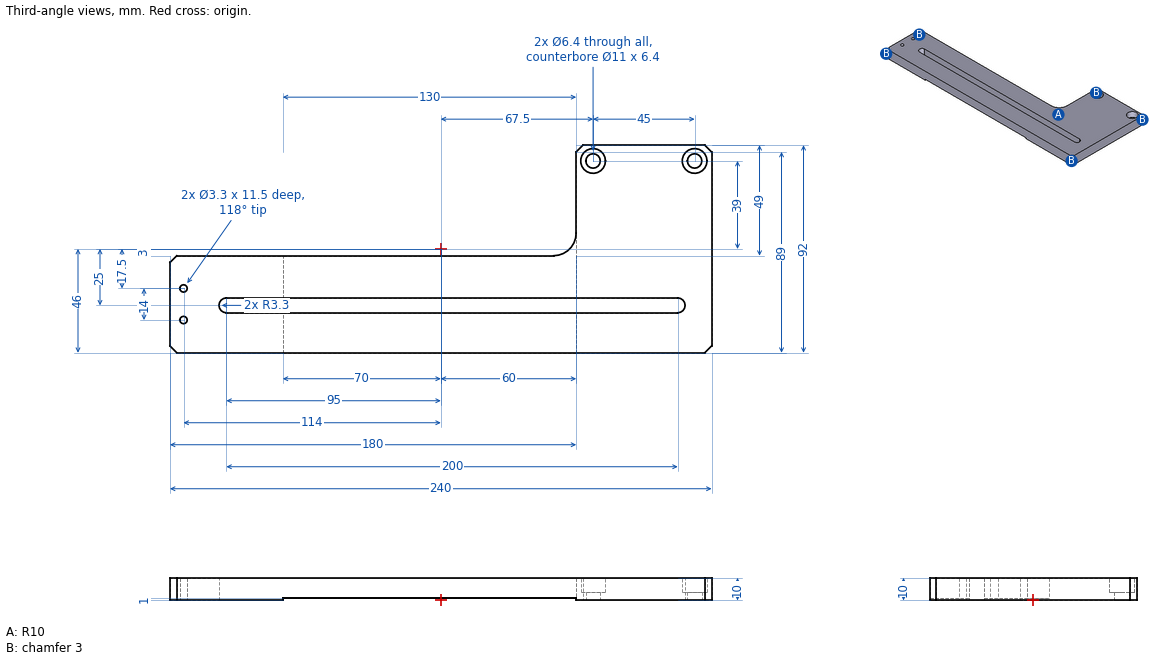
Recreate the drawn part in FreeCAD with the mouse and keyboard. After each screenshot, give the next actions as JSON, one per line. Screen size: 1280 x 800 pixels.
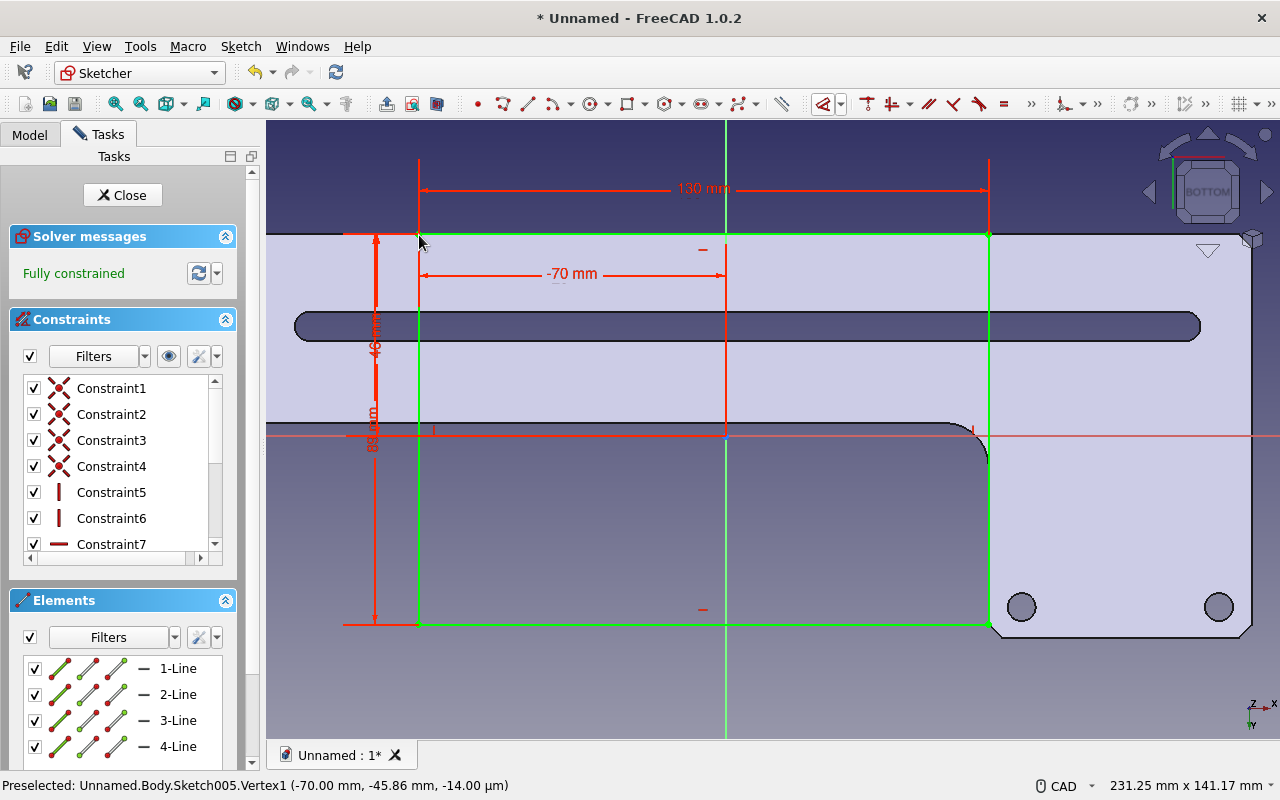
{"action": "left_click", "coordinate": [123, 195]}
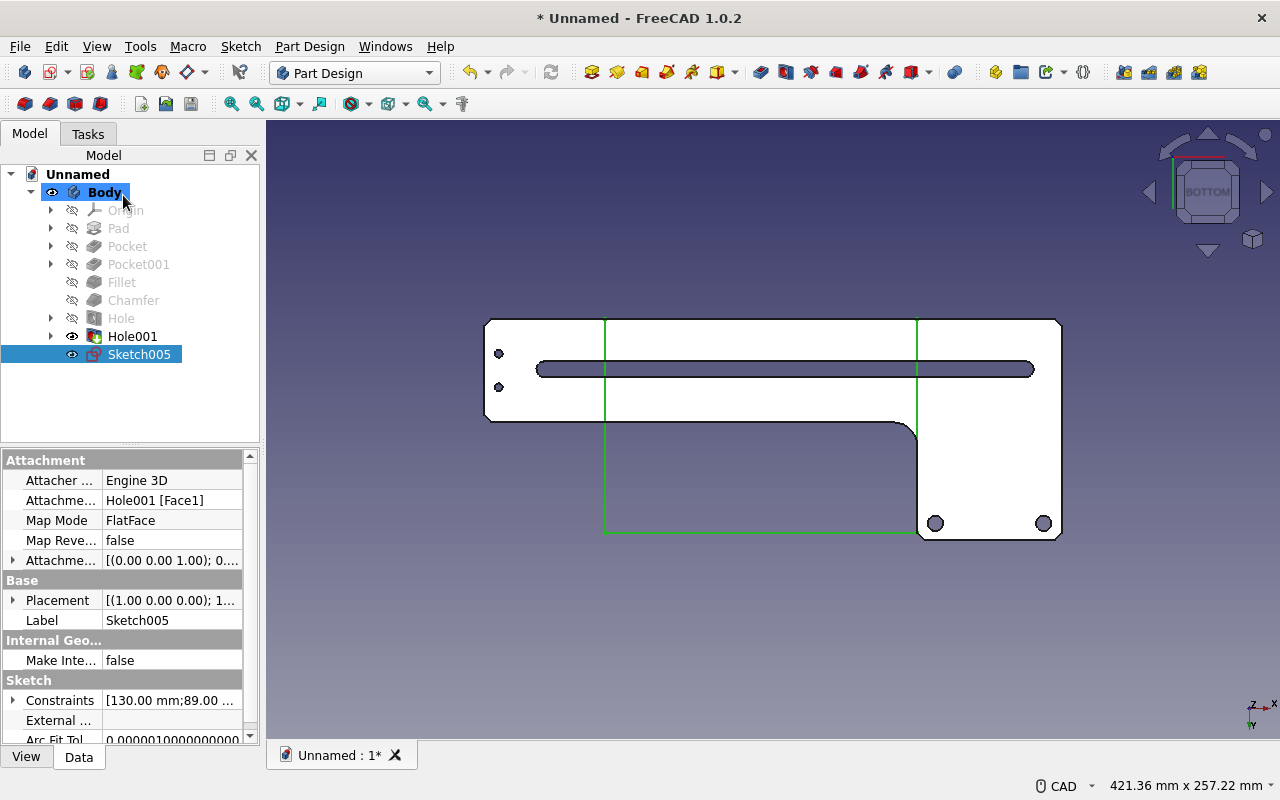
{"action": "left_click", "coordinate": [761, 72]}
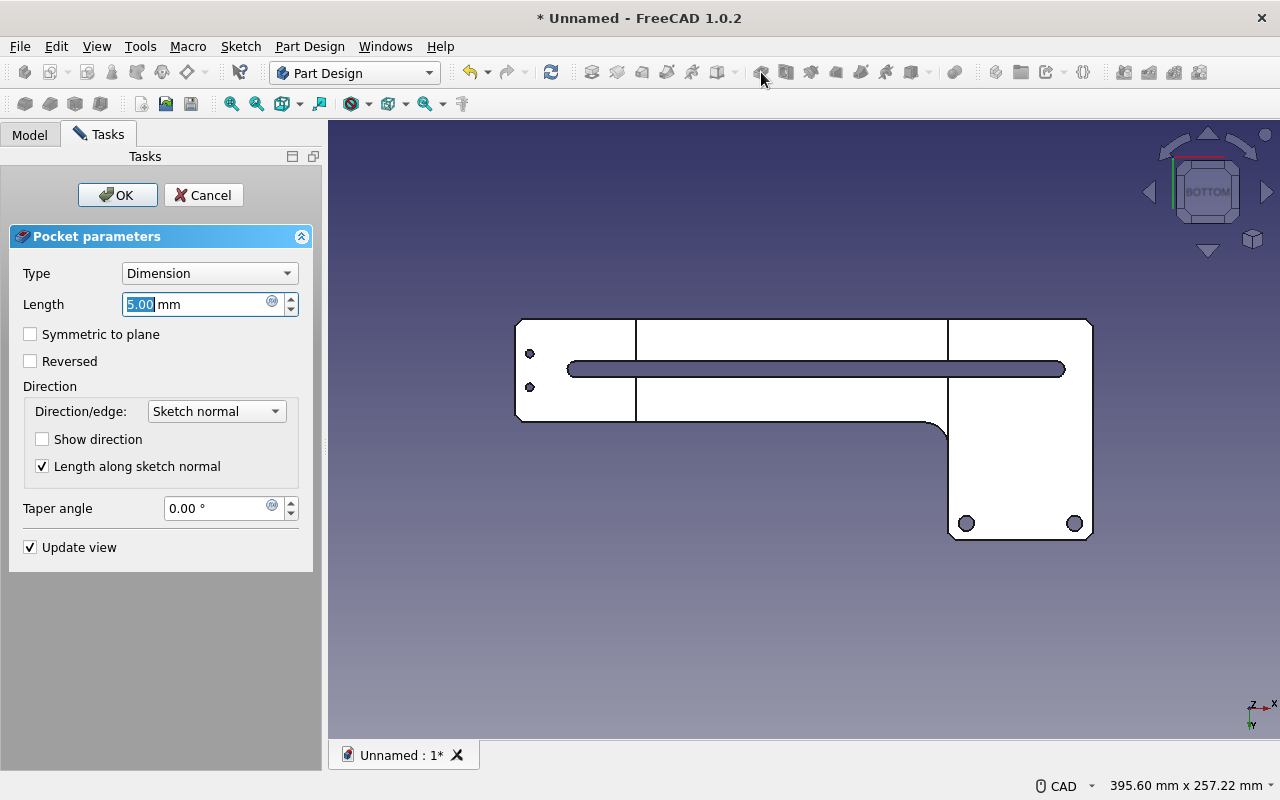
{"action": "type", "text": "1"}
{"action": "key", "text": "Tab"}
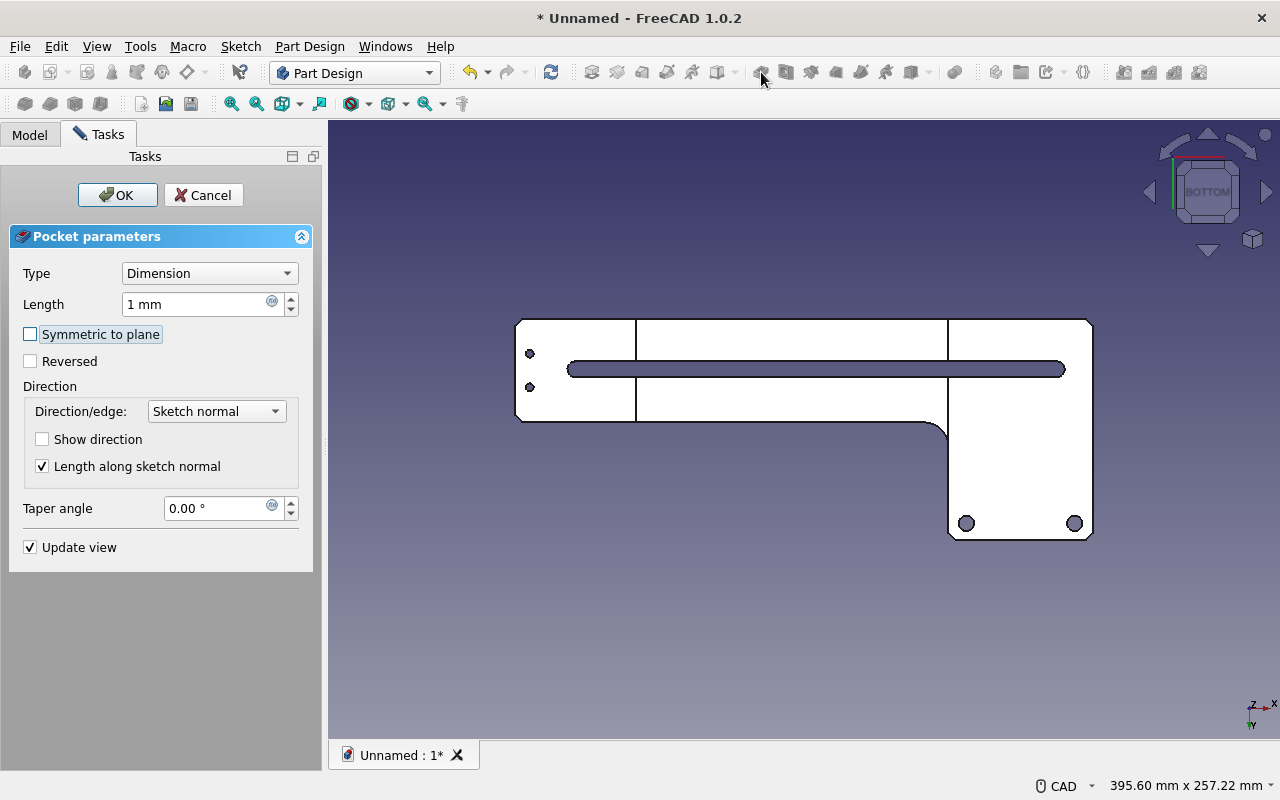
{"action": "left_click", "coordinate": [118, 195]}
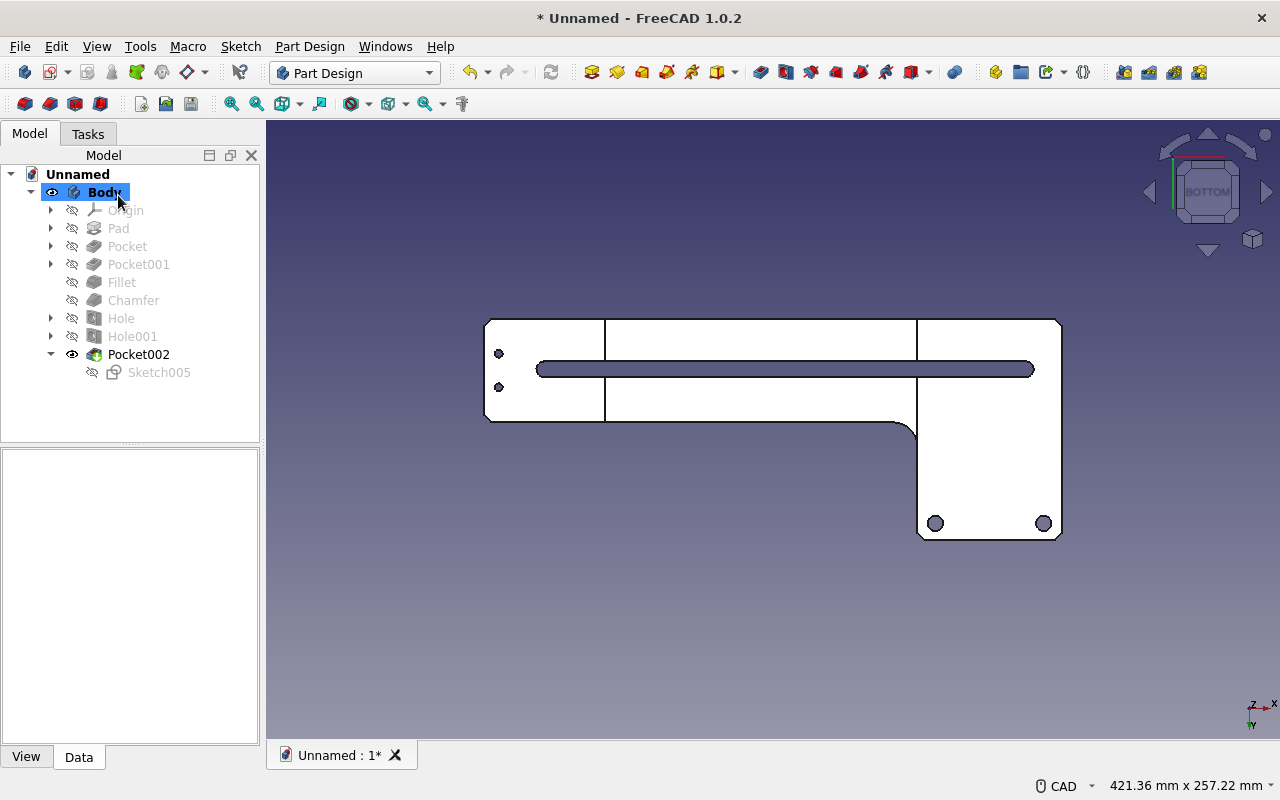
{"action": "key", "text": "0"}